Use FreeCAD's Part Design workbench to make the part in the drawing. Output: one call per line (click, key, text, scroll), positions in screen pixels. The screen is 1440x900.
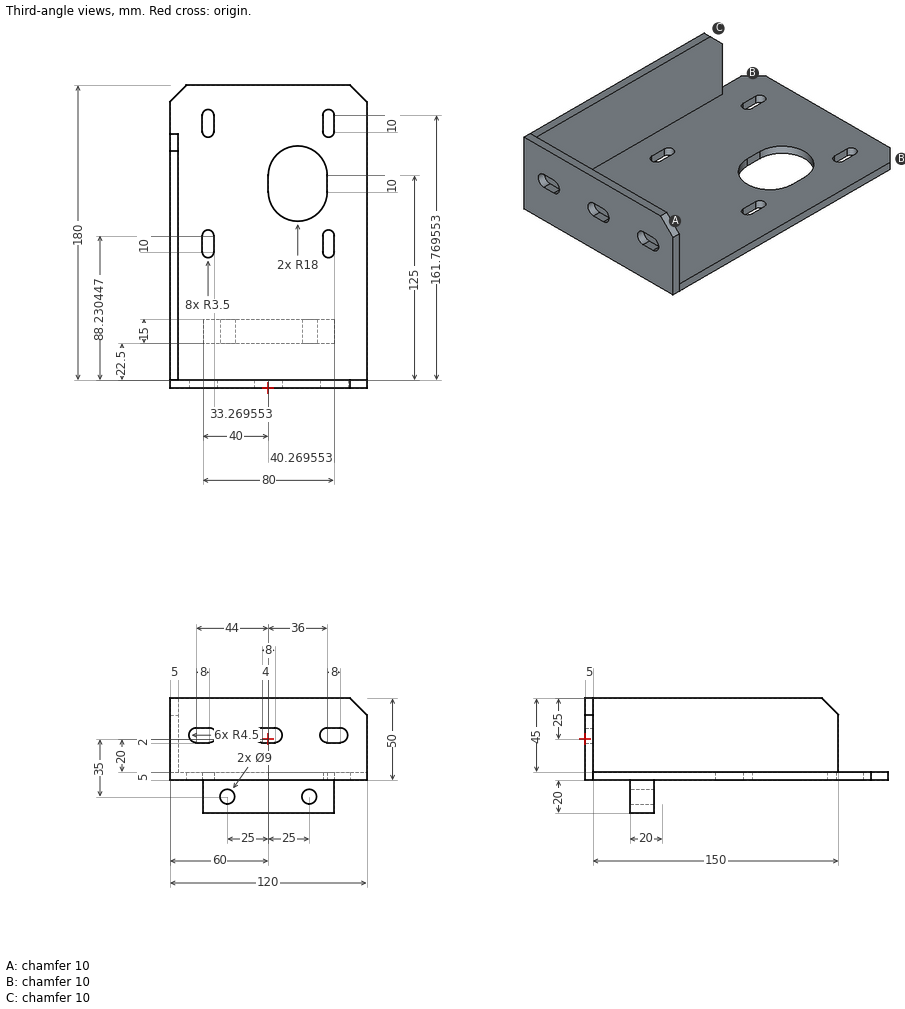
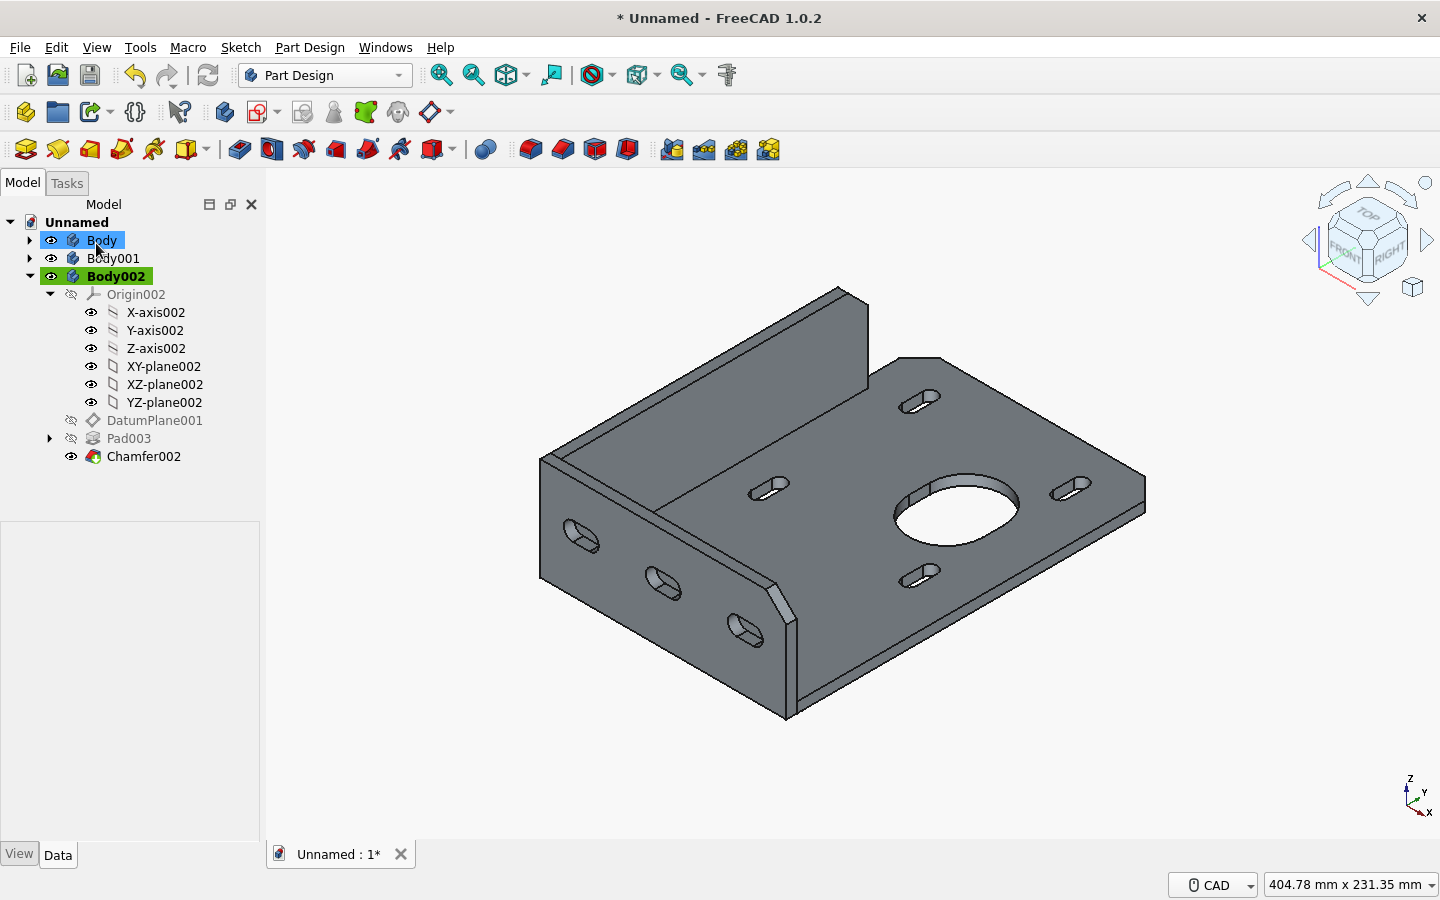
key(v)
key(f)